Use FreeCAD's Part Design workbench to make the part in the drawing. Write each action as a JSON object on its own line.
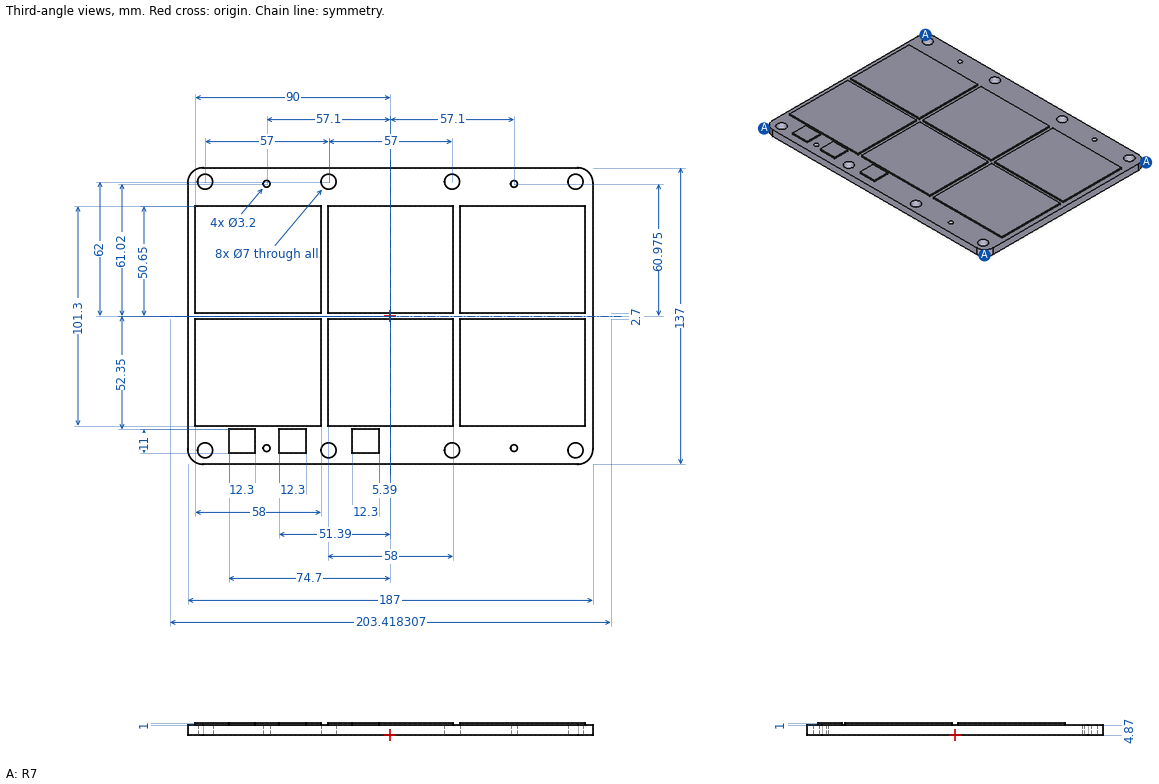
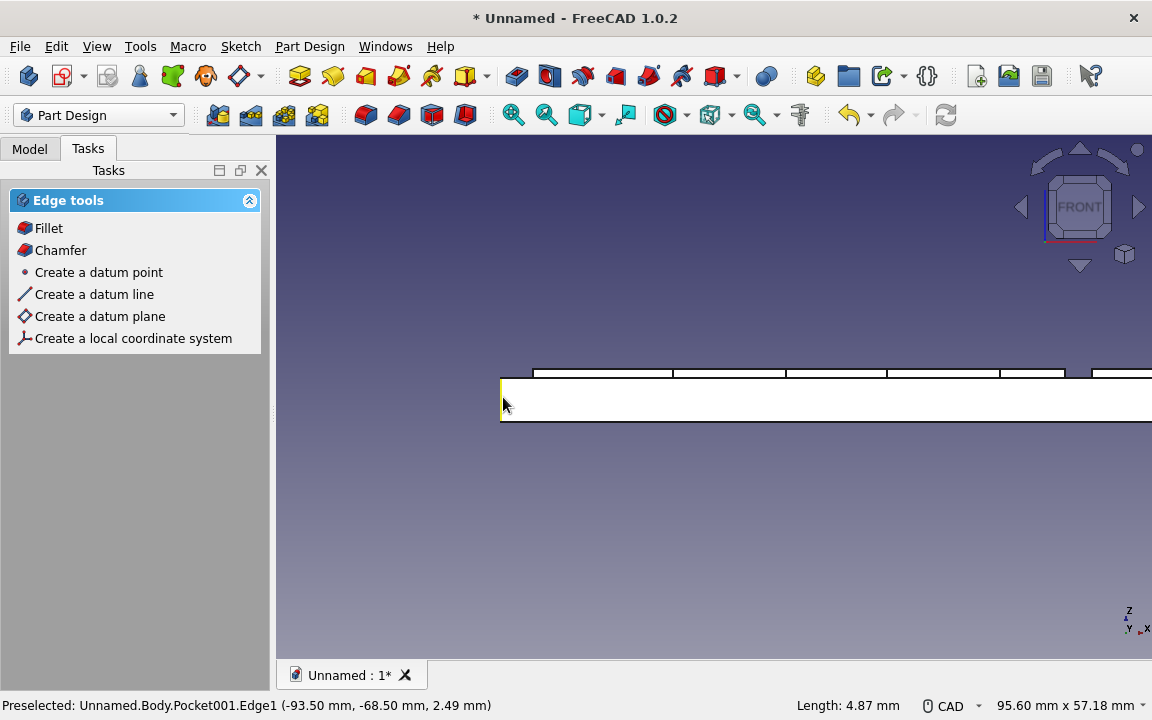
{"action": "left_click", "coordinate": [501, 399], "text": "ctrl"}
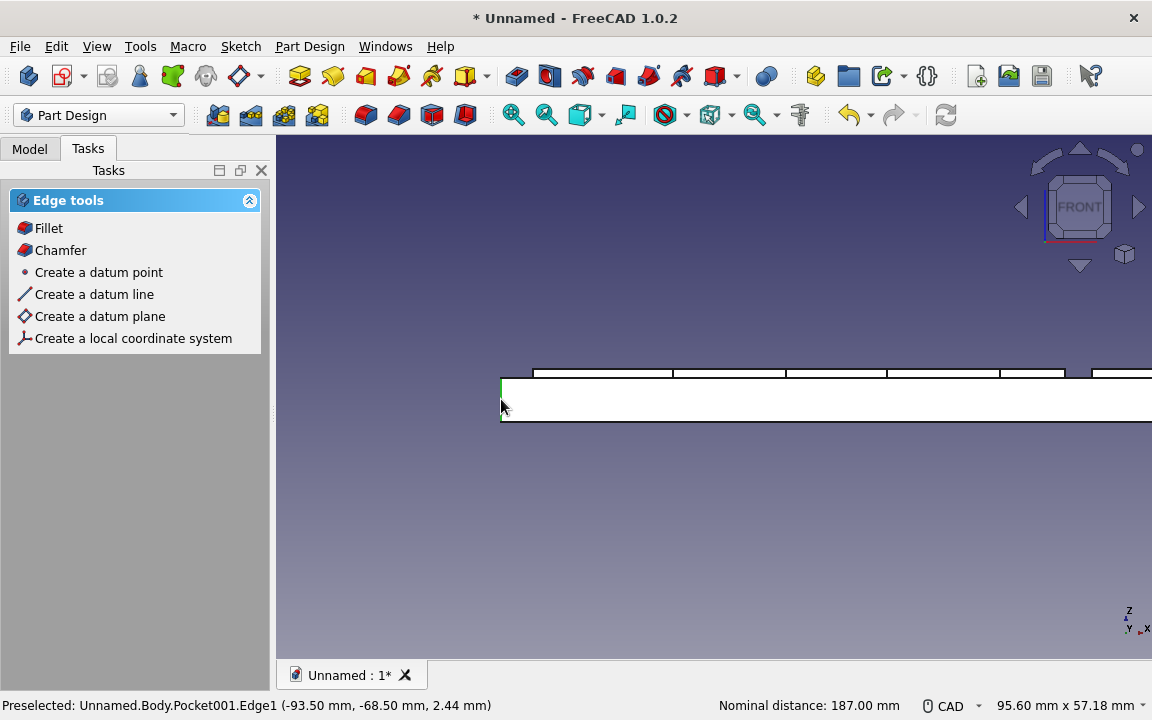
{"action": "left_click", "coordinate": [514, 116]}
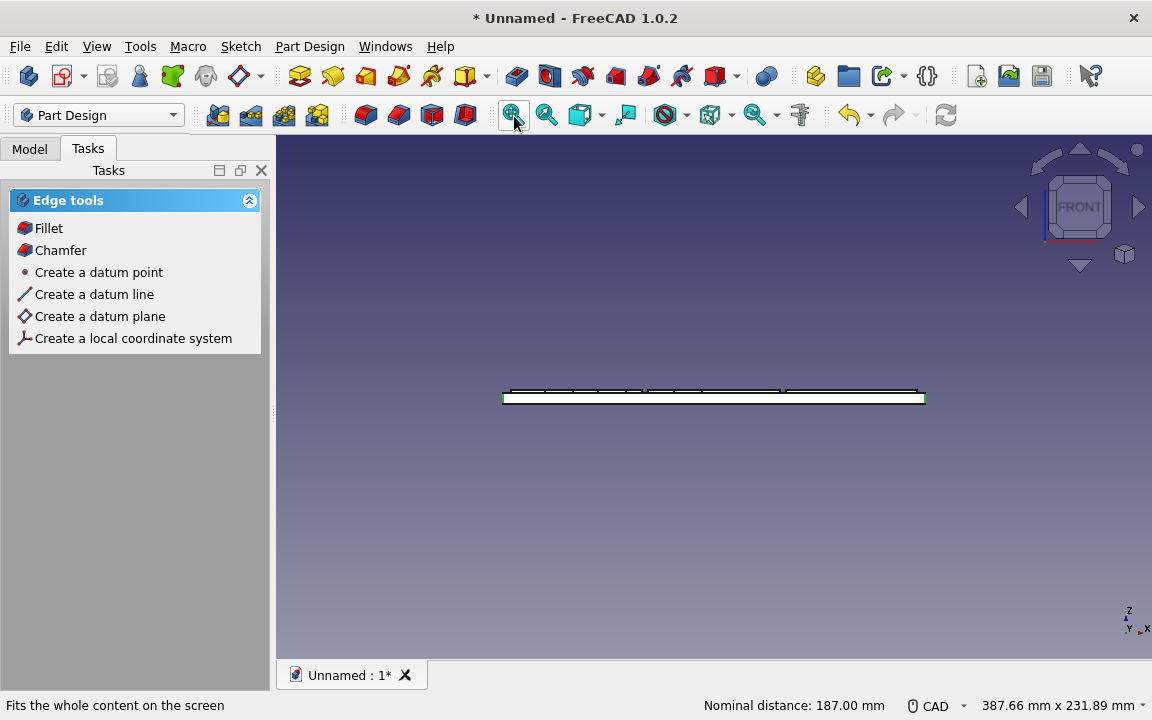
{"action": "key", "text": "3"}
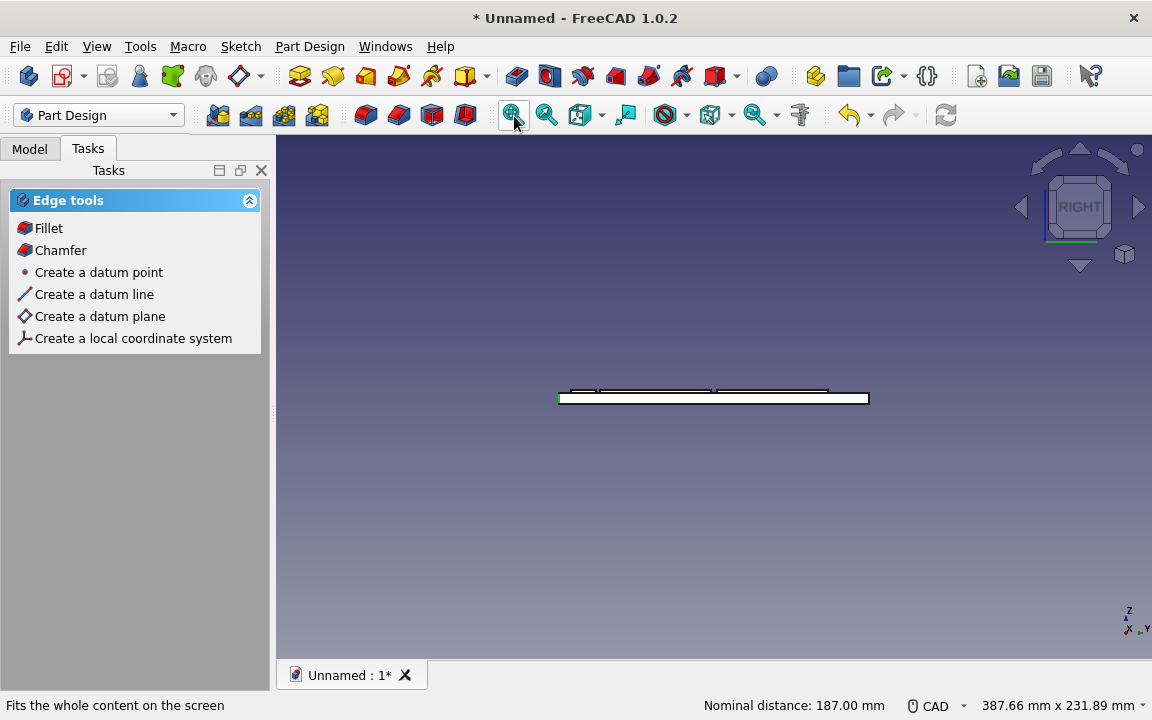
{"action": "key", "text": "v f"}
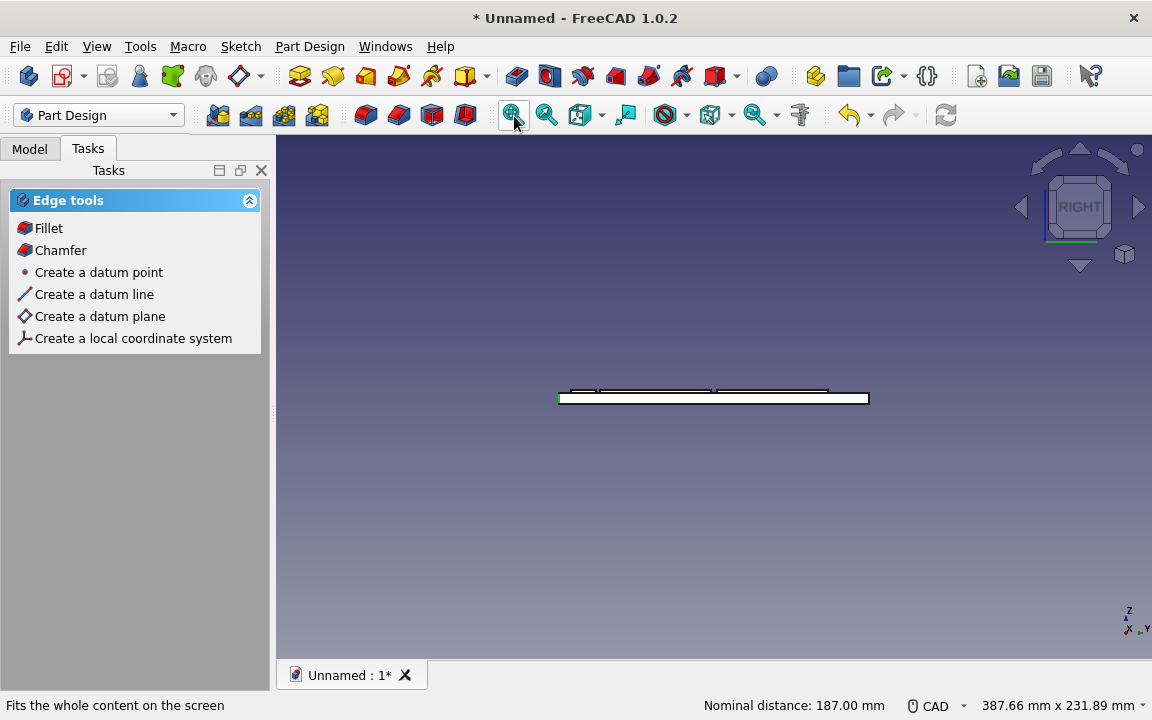
{"action": "scroll", "coordinate": [869, 397], "scroll_direction": "up", "scroll_amount": 7}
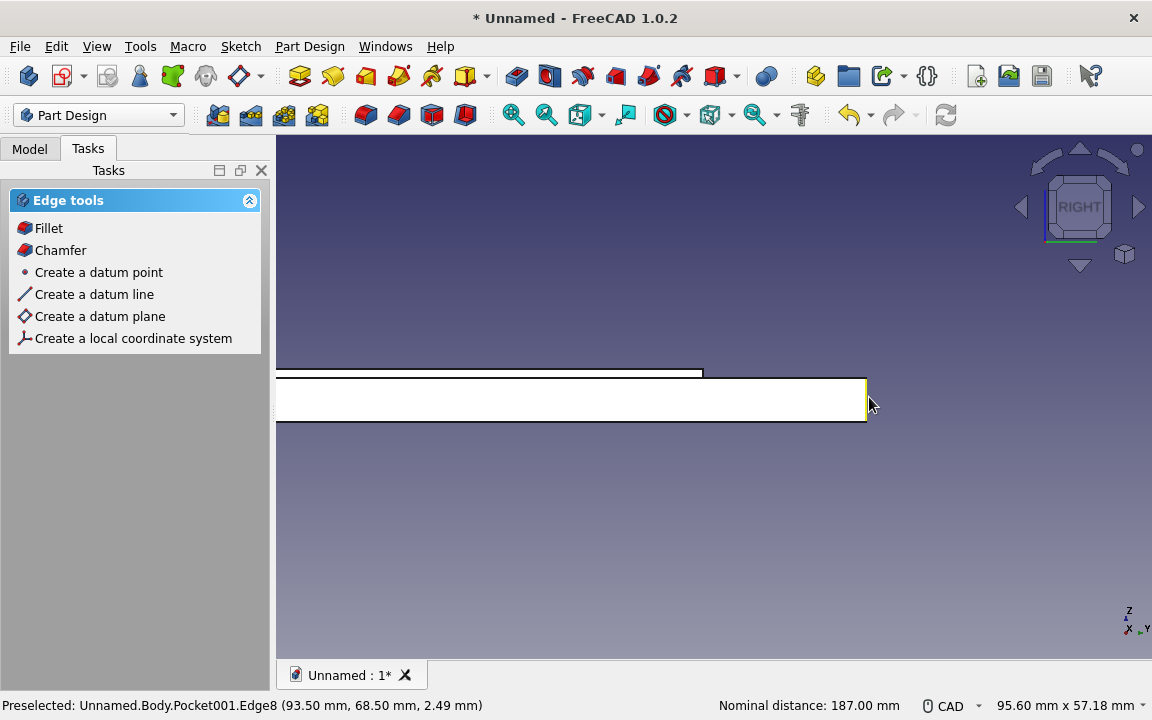
{"action": "left_click", "coordinate": [866, 399], "text": "ctrl"}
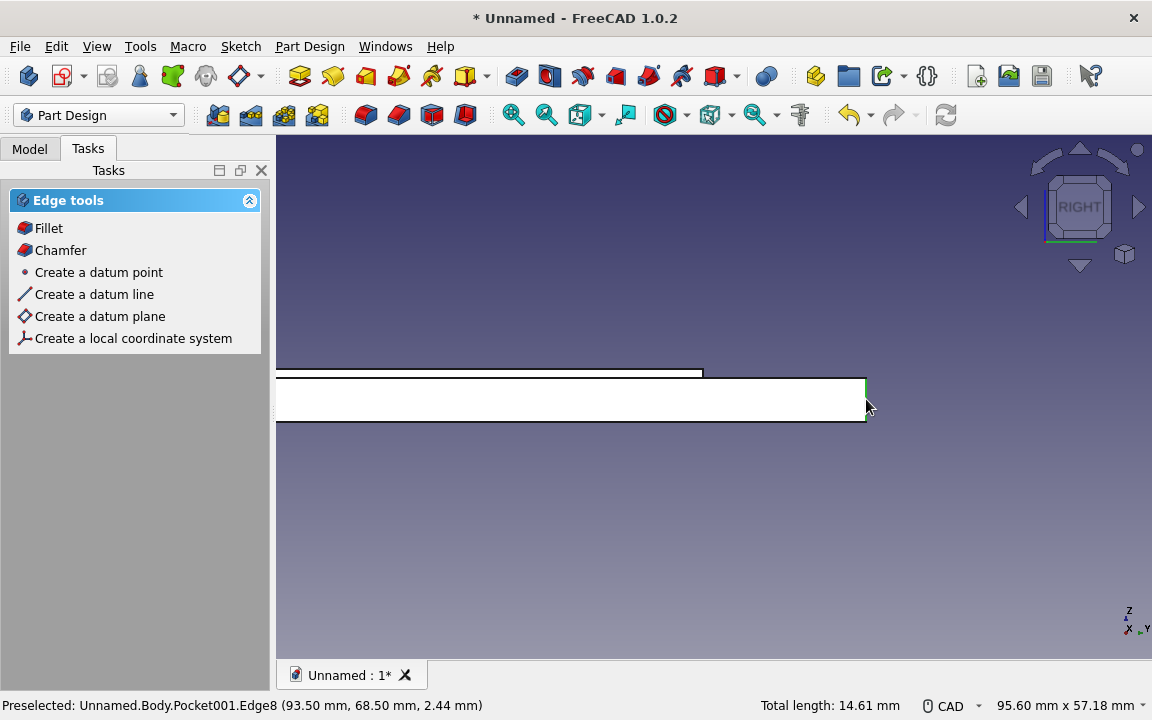
{"action": "key", "text": "v f"}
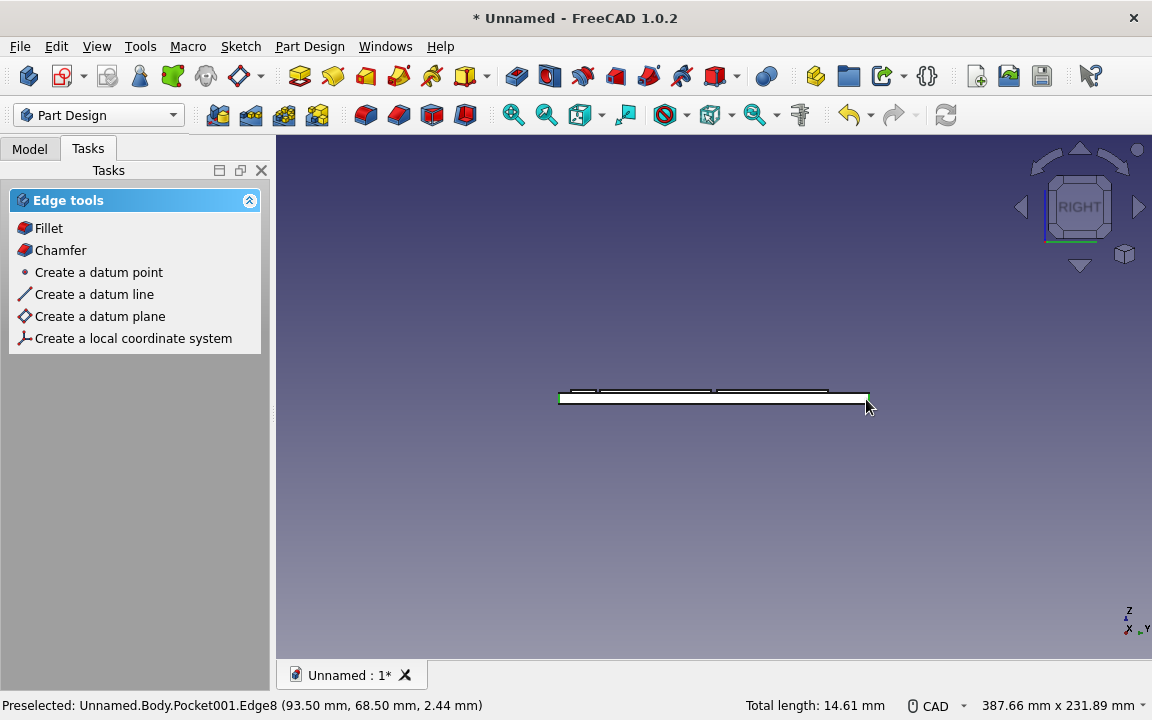
{"action": "key", "text": "5"}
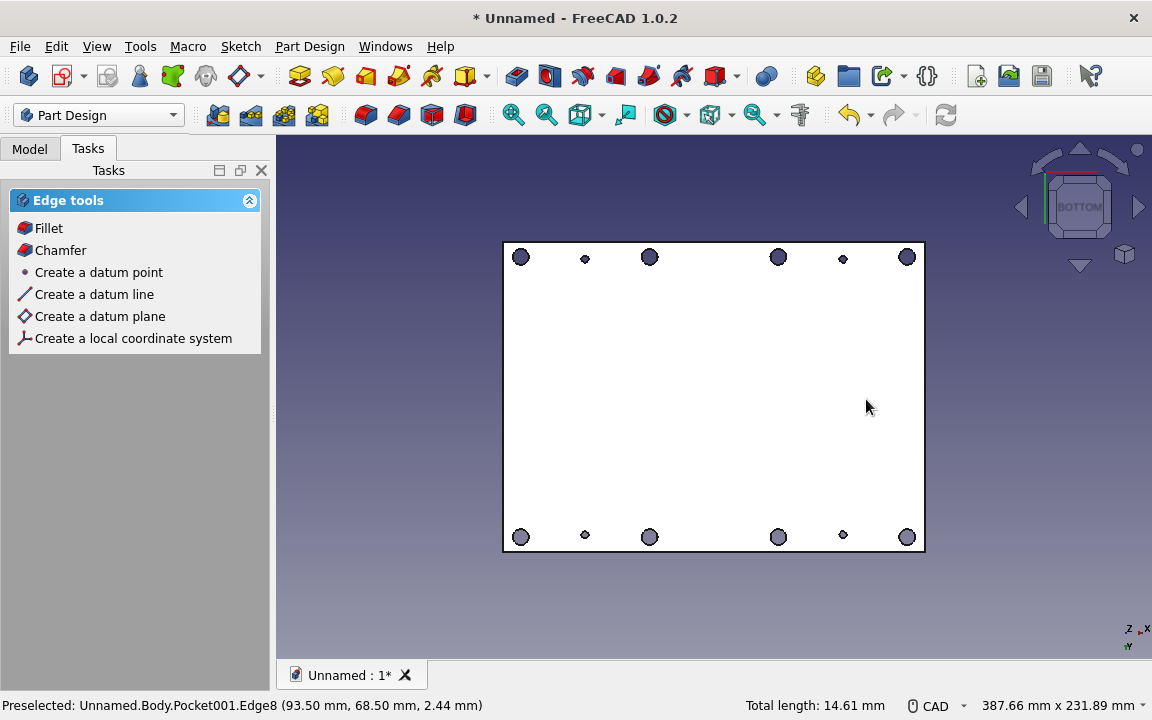
{"action": "scroll", "coordinate": [503, 551], "scroll_direction": "up", "scroll_amount": 7}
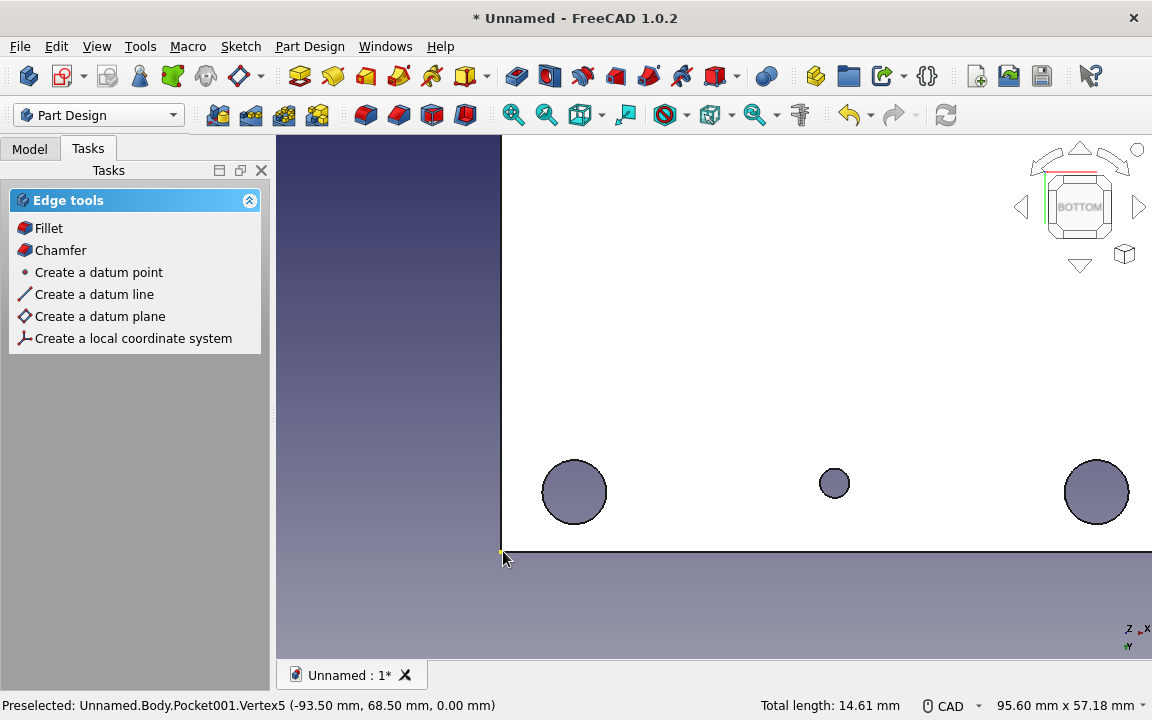
{"action": "key", "text": "v f"}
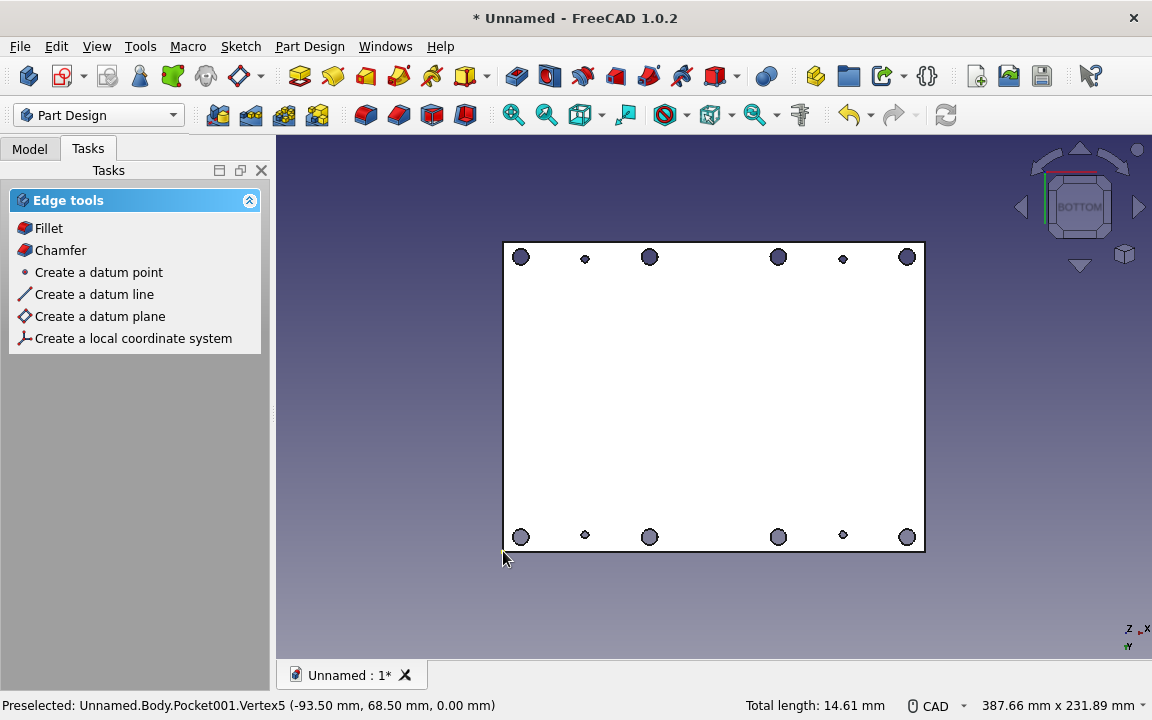
{"action": "key", "text": "4"}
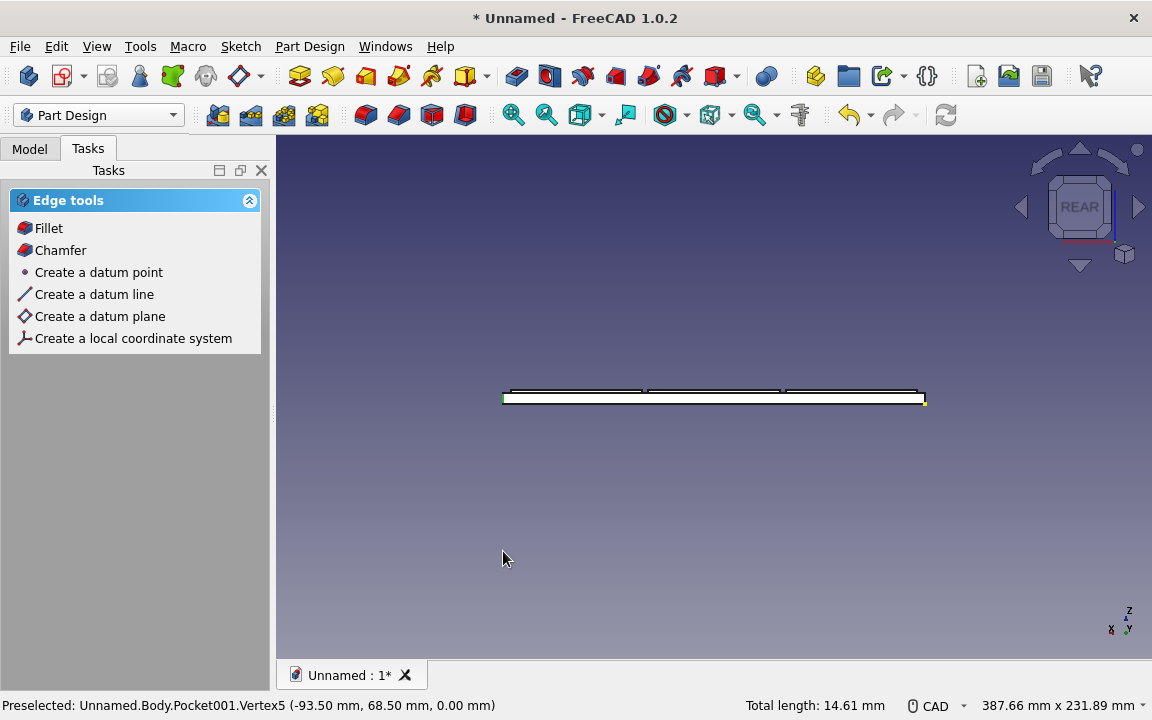
{"action": "scroll", "coordinate": [925, 397], "scroll_direction": "up", "scroll_amount": 7}